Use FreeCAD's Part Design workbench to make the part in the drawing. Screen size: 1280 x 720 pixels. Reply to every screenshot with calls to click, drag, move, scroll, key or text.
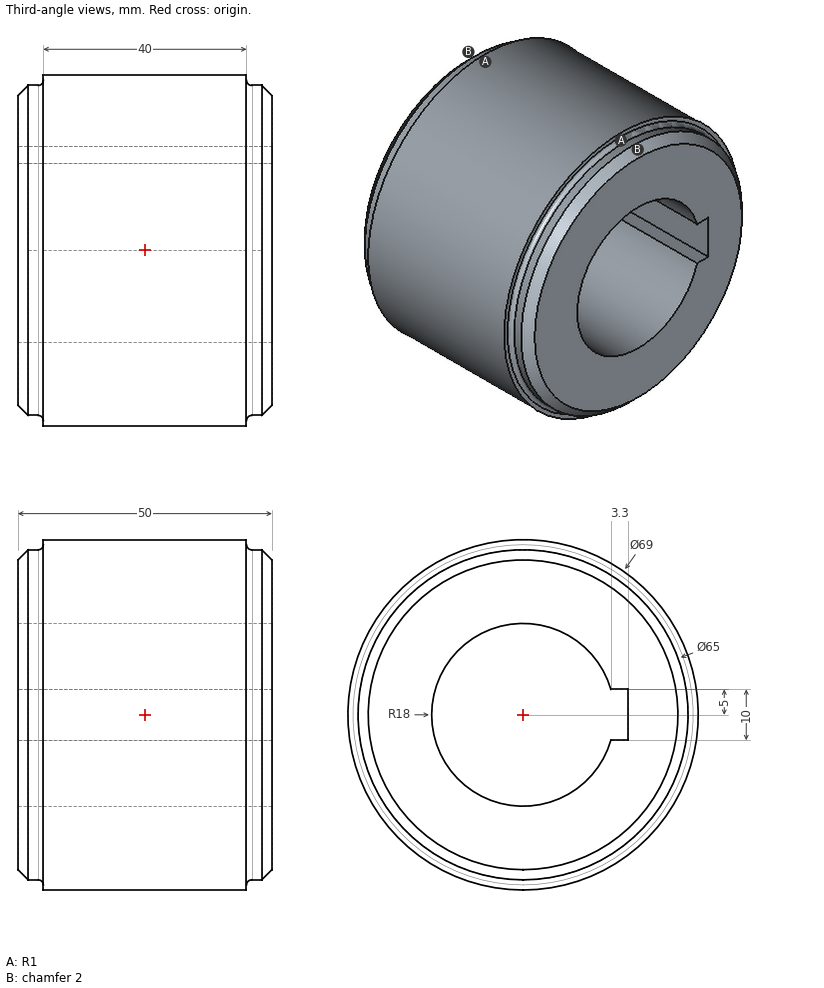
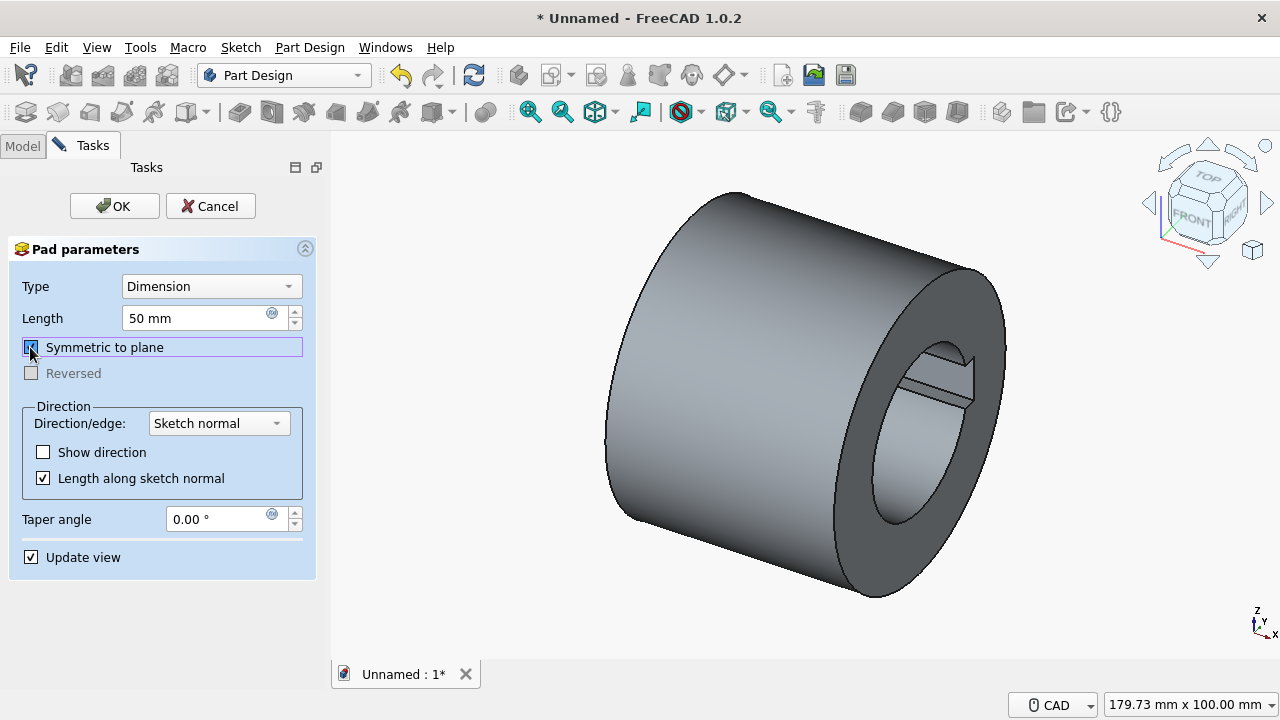
click(115, 206)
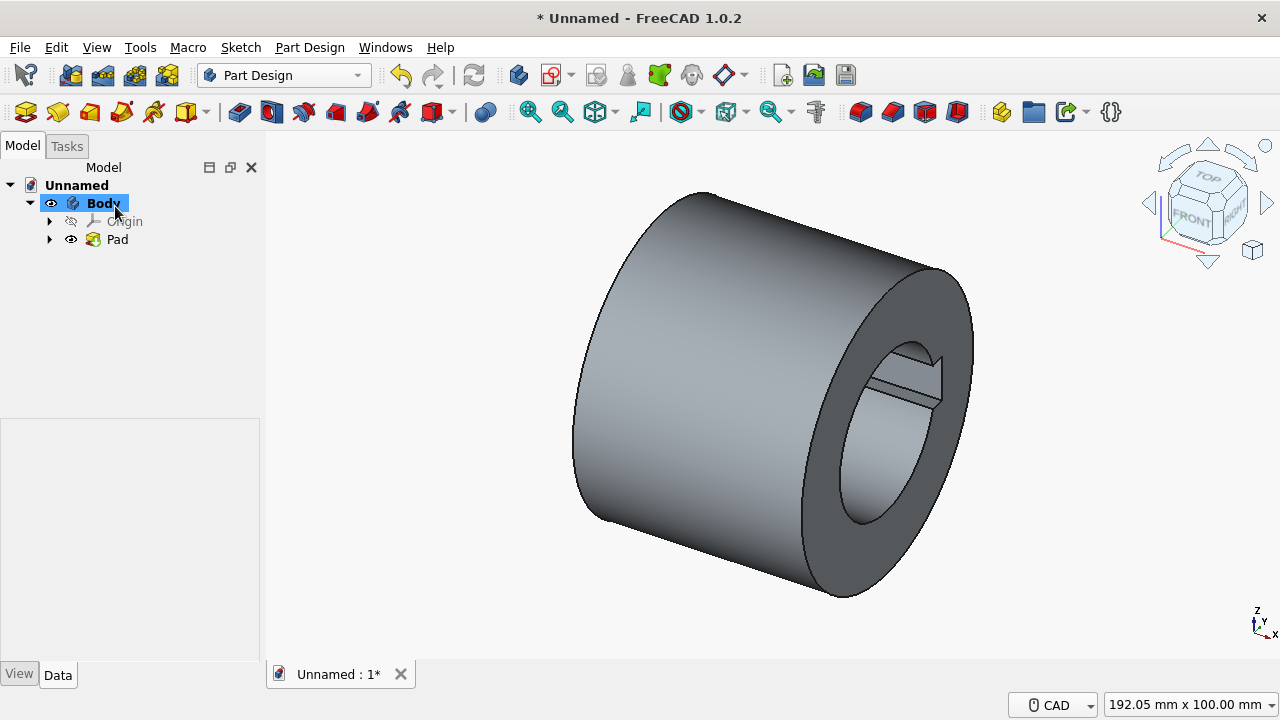
key(v)
key(f)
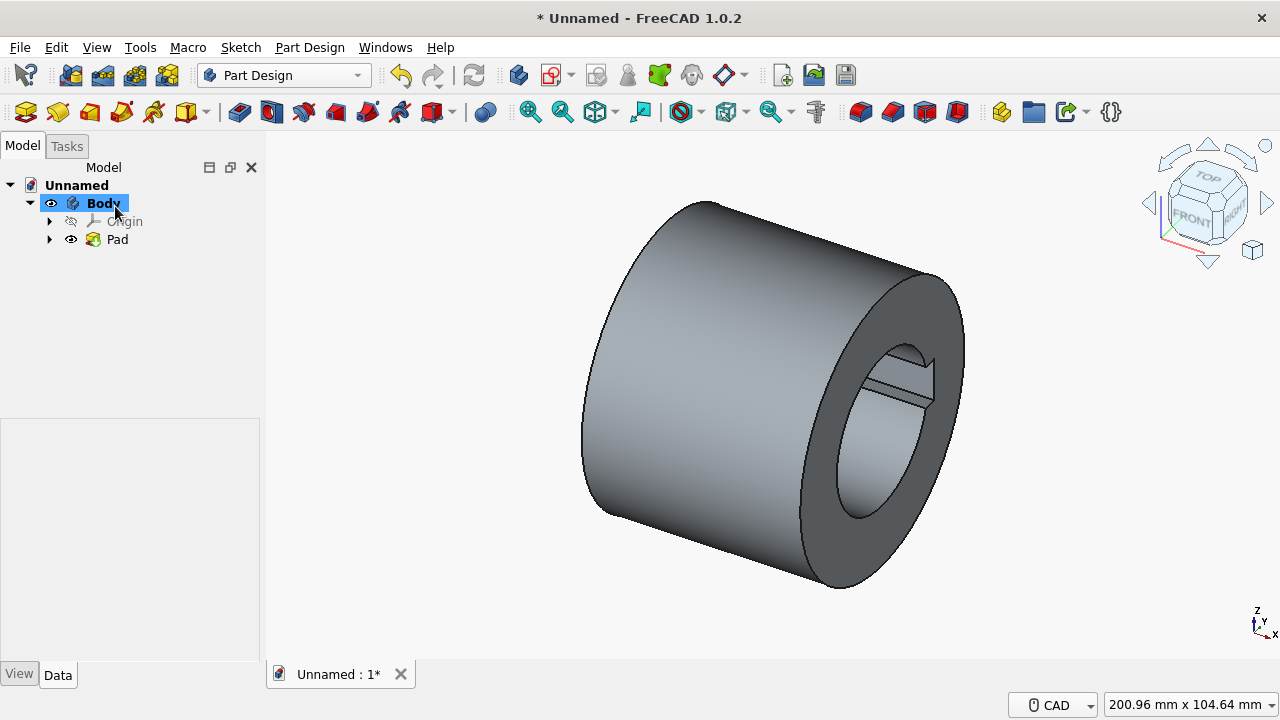
click(552, 76)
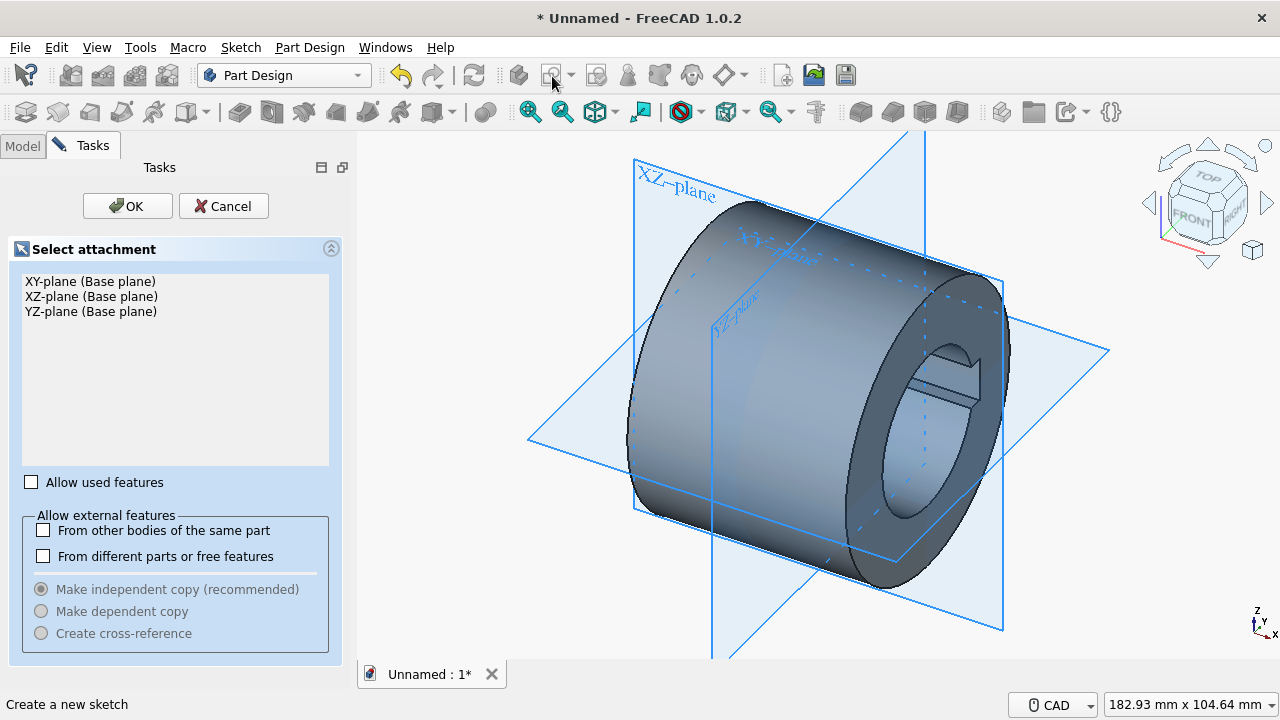
click(82, 312)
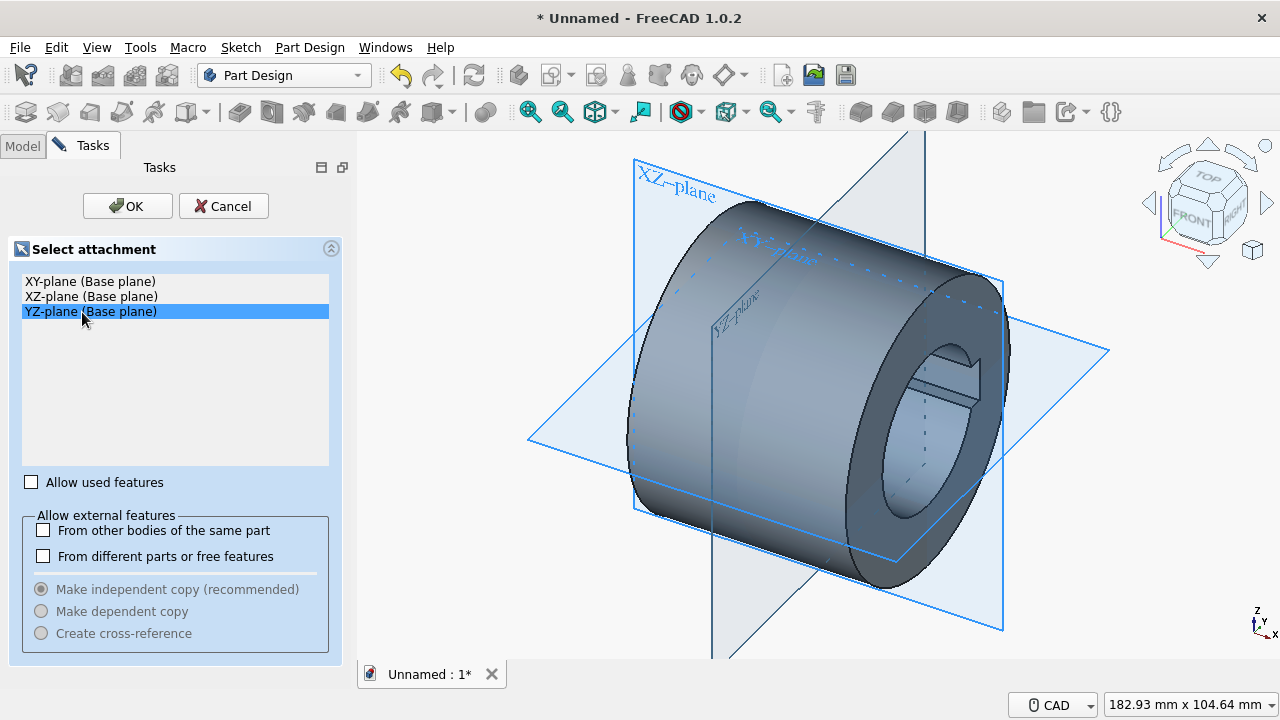
click(128, 206)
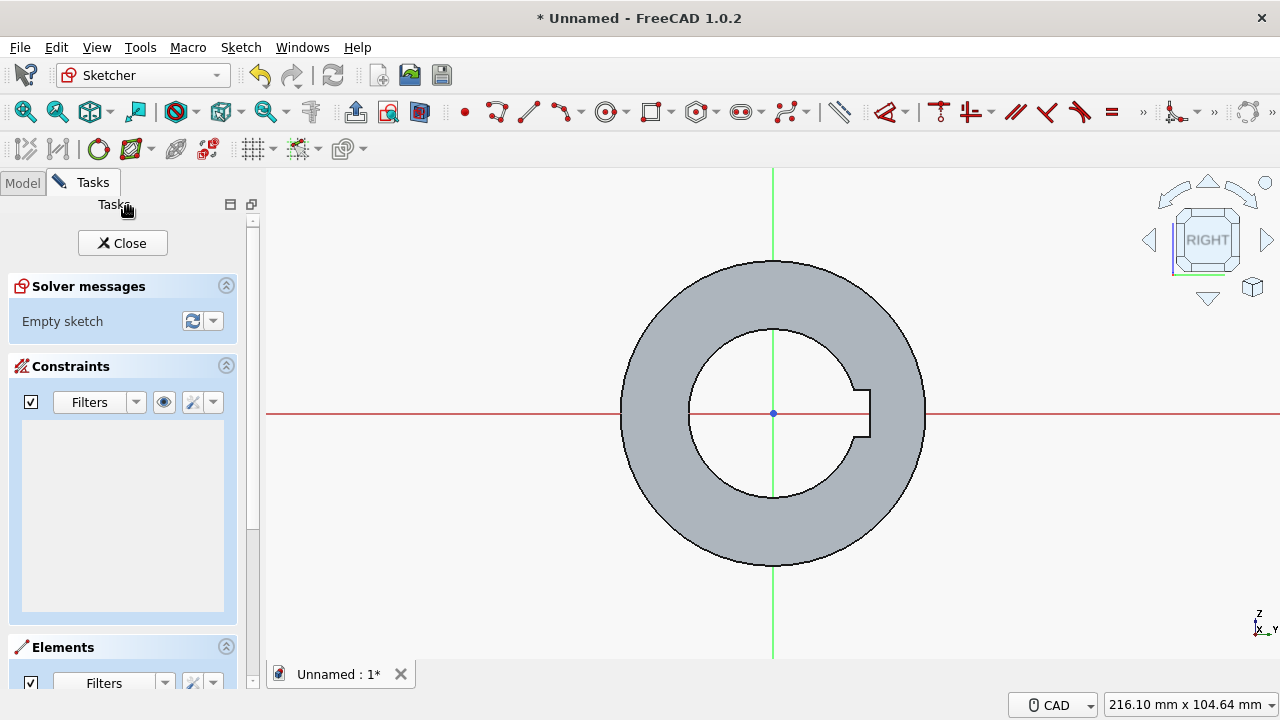
key(q)
key(s)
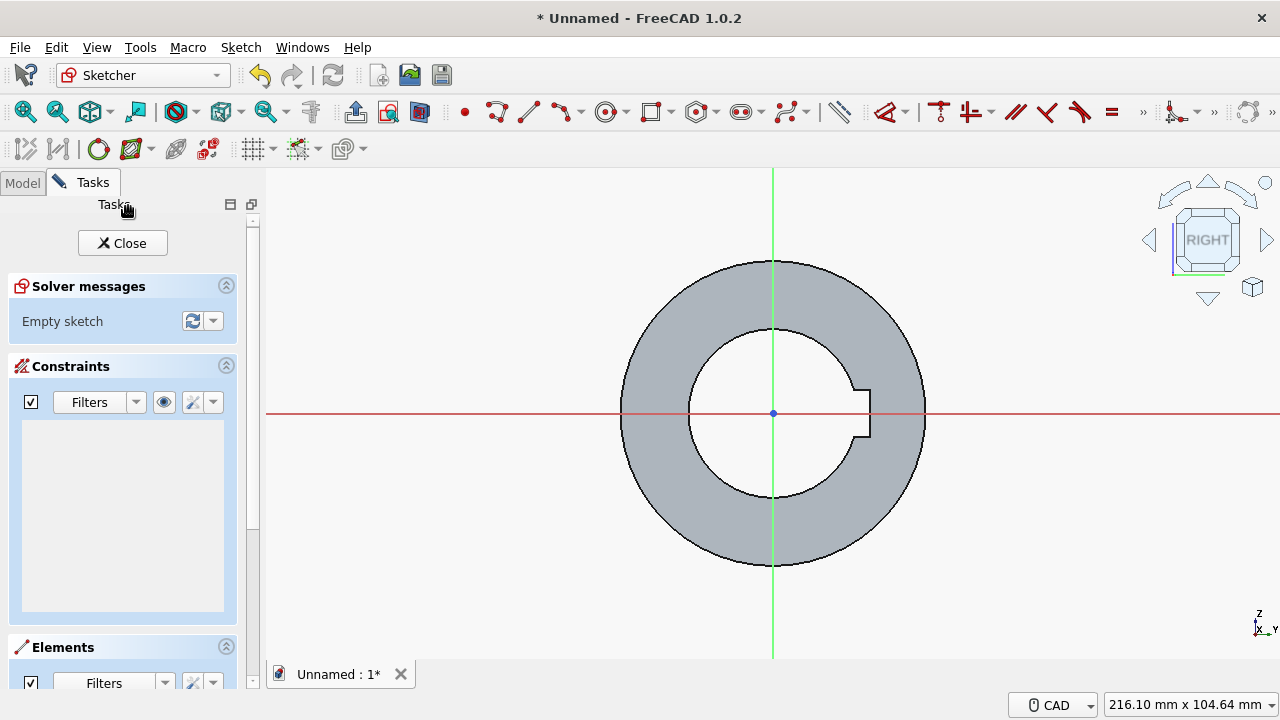
click(606, 112)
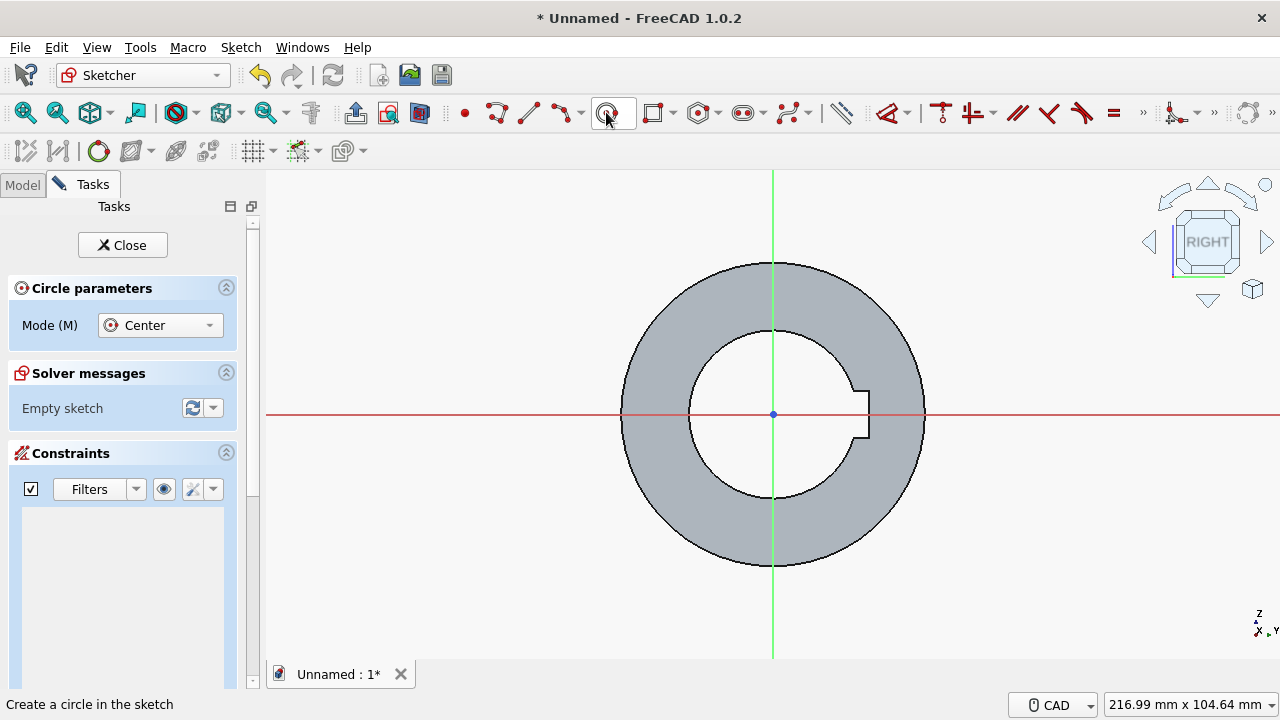
click(773, 414)
move(887, 300)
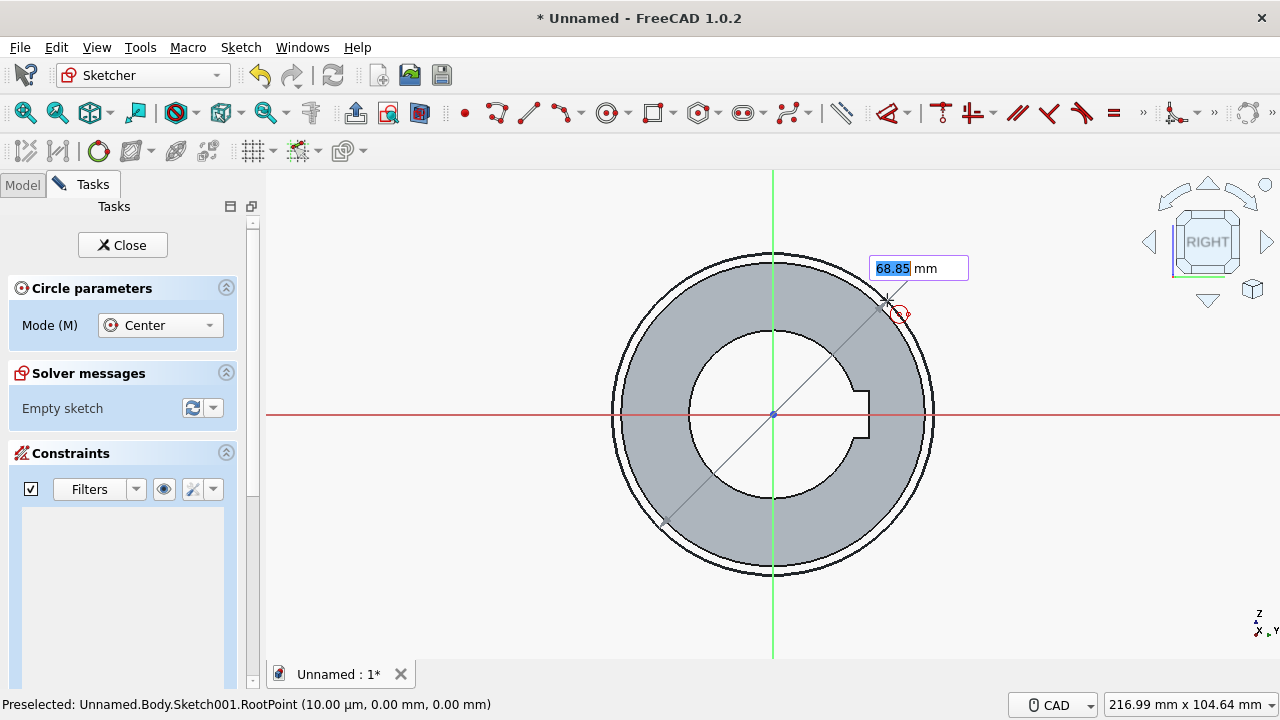
text(69)
key(Return)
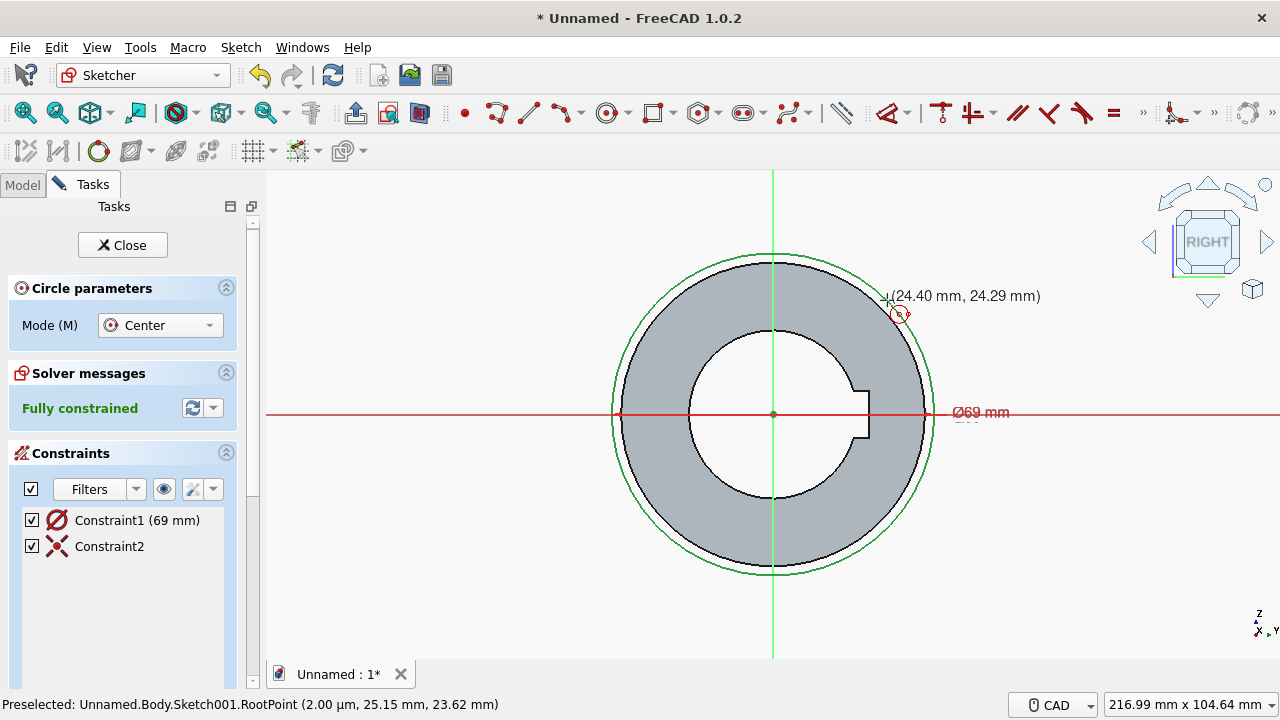
click(773, 414)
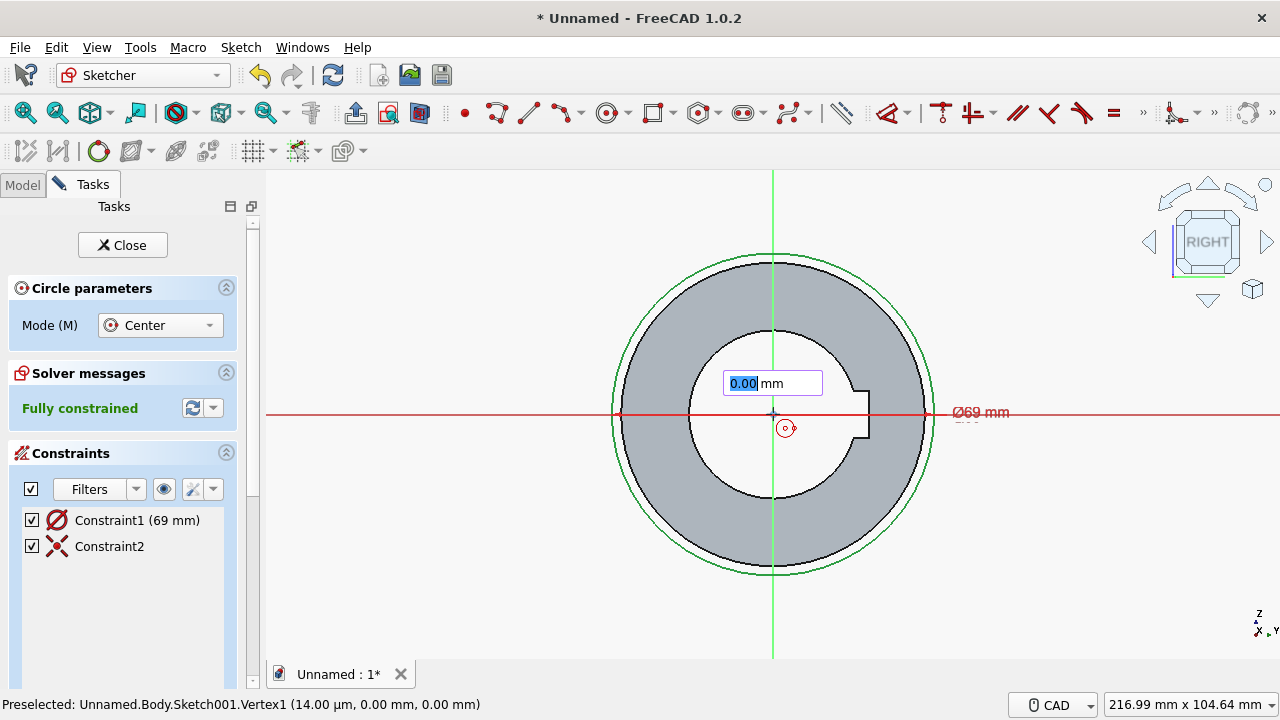
scroll(880, 307, up, 3)
move(880, 307)